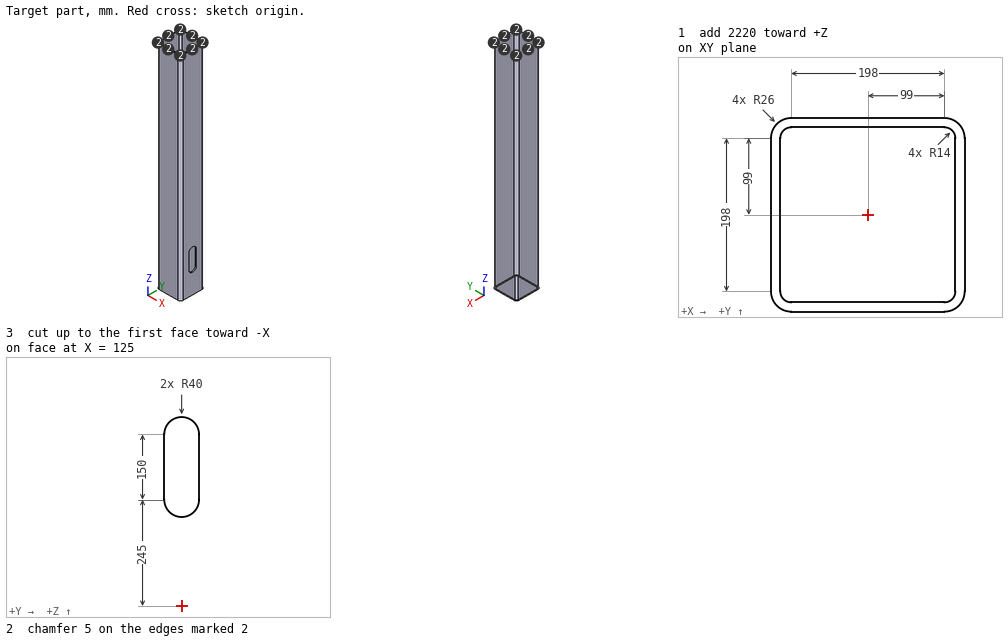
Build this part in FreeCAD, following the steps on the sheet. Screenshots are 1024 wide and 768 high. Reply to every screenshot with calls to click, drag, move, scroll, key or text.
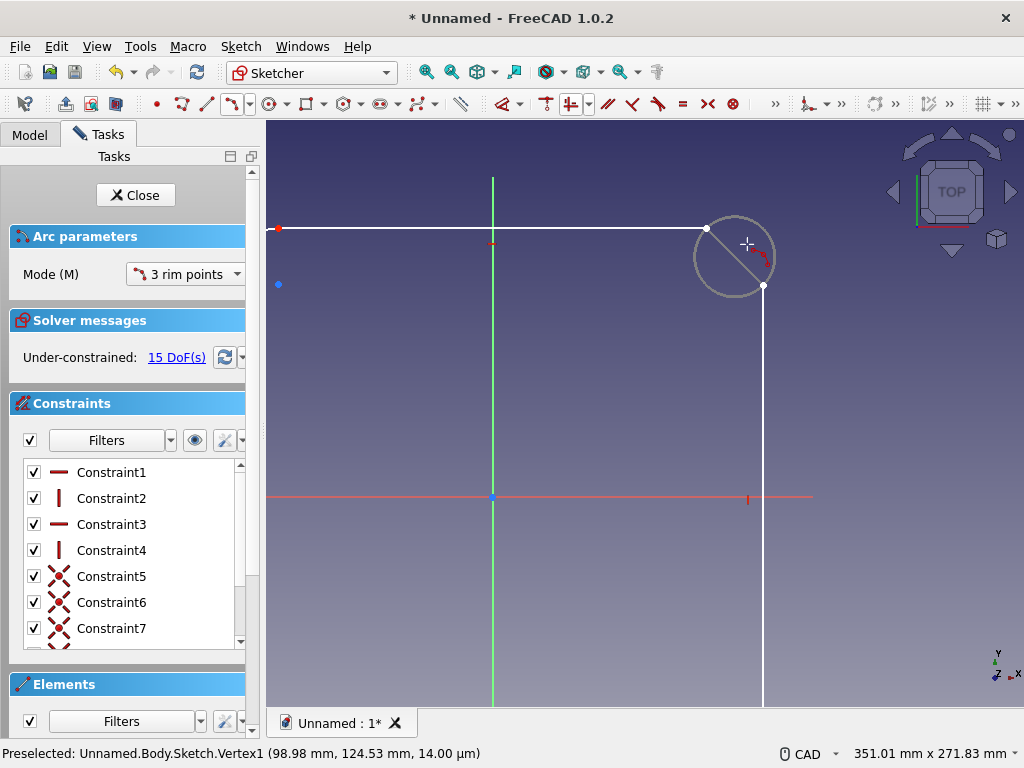
click(746, 244)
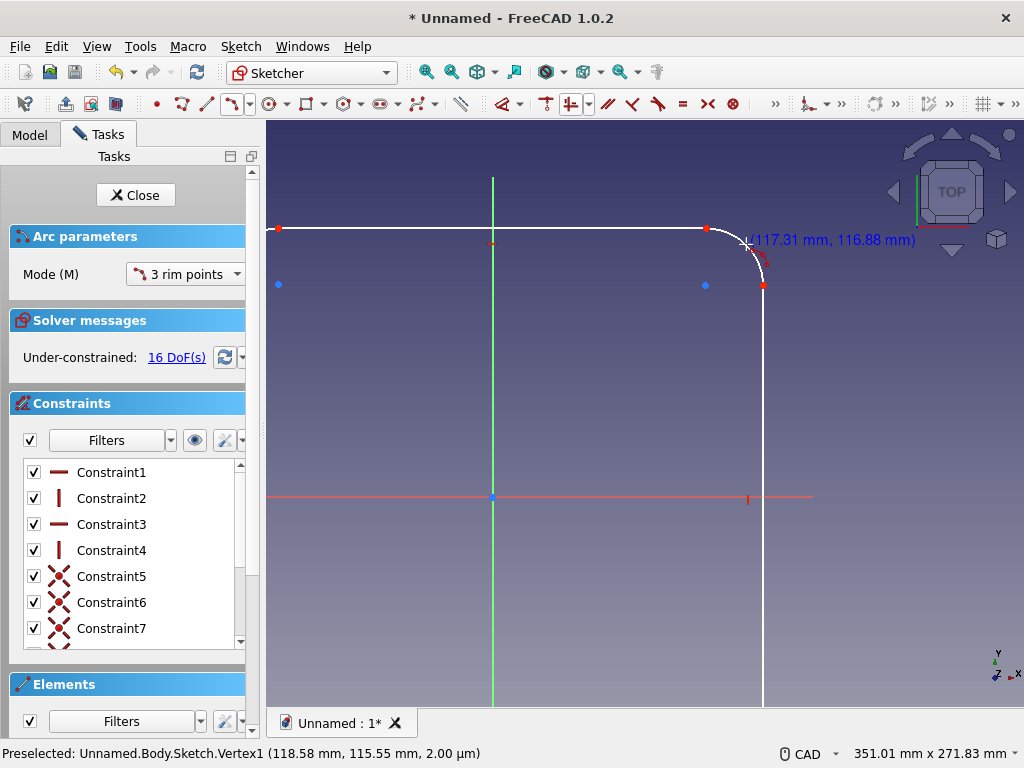
click(207, 104)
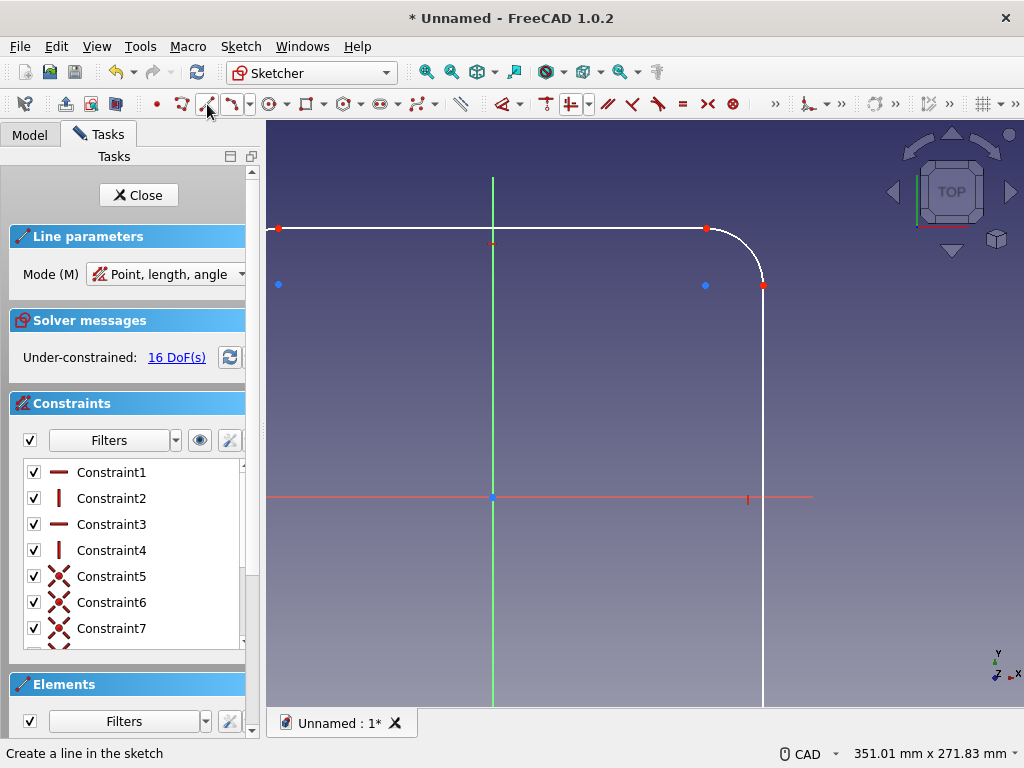
scroll(747, 243, down, 2)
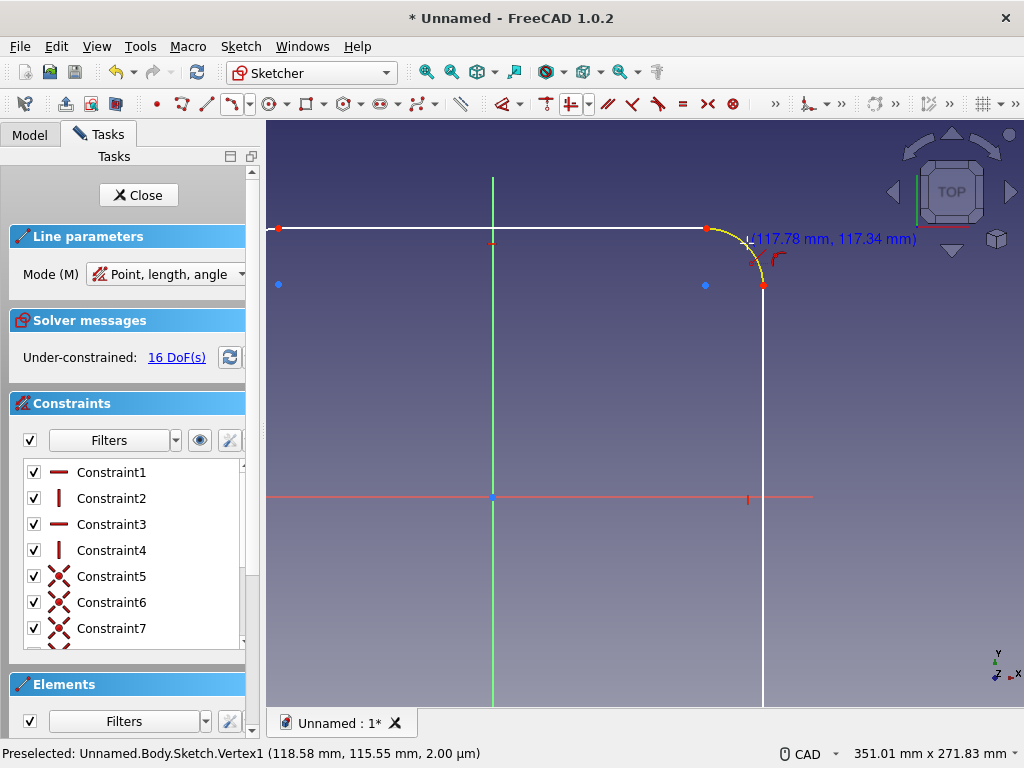
click(433, 250)
click(720, 250)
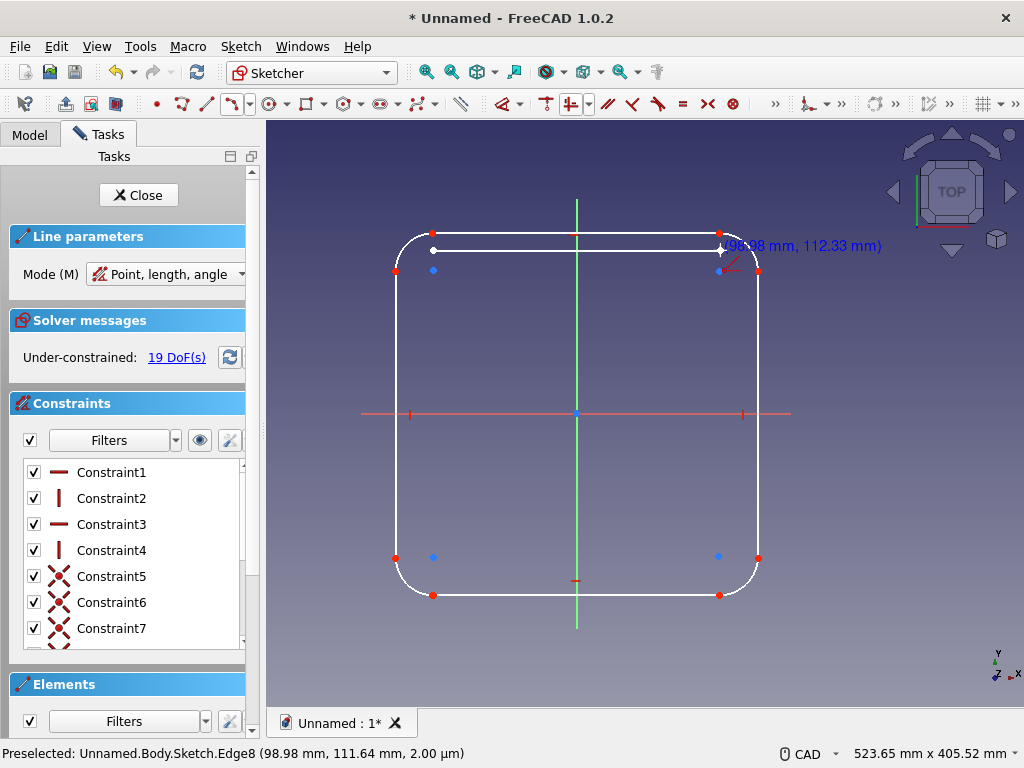
click(740, 270)
click(740, 557)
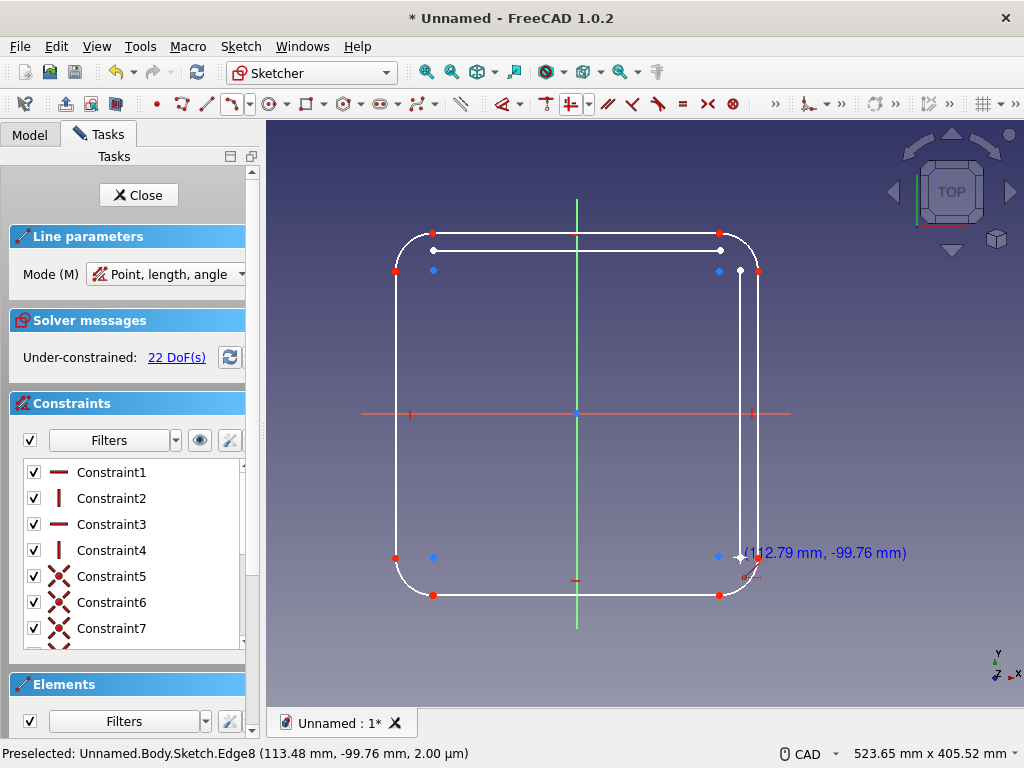
click(720, 577)
click(433, 577)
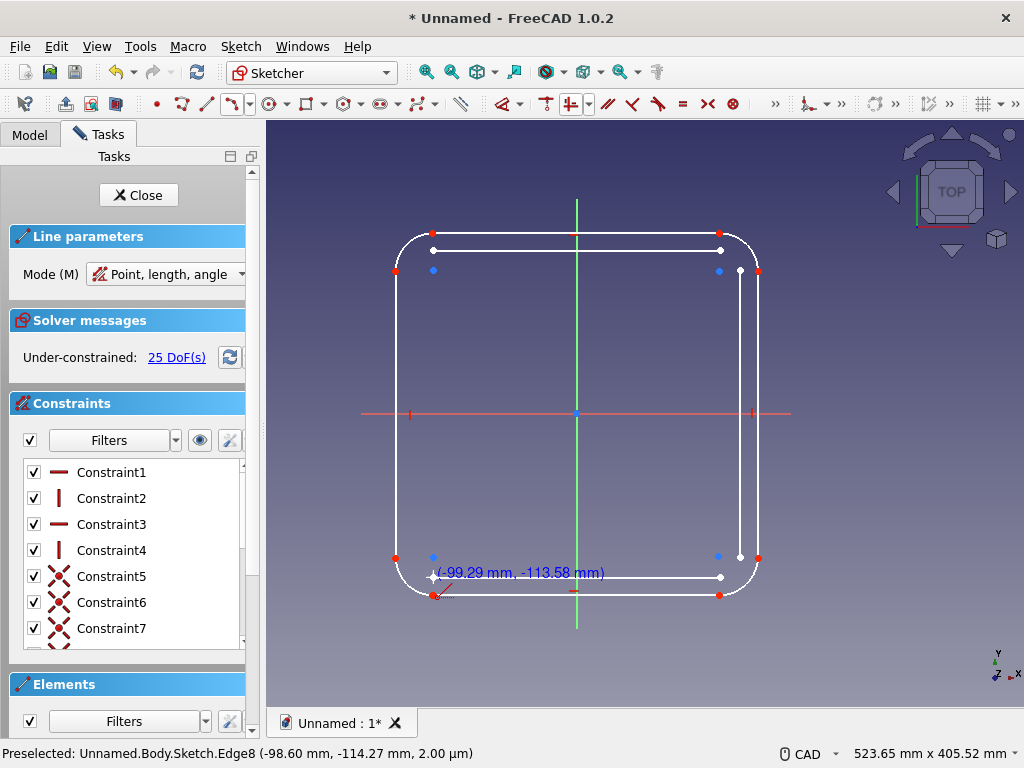
click(413, 557)
click(413, 270)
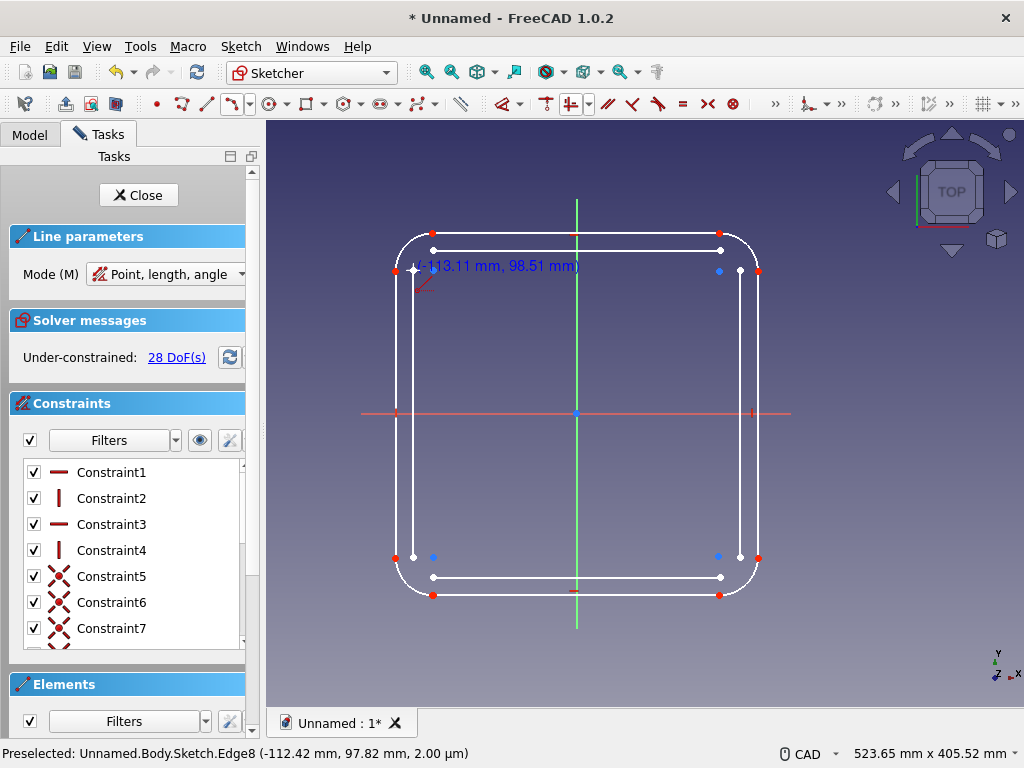
click(232, 104)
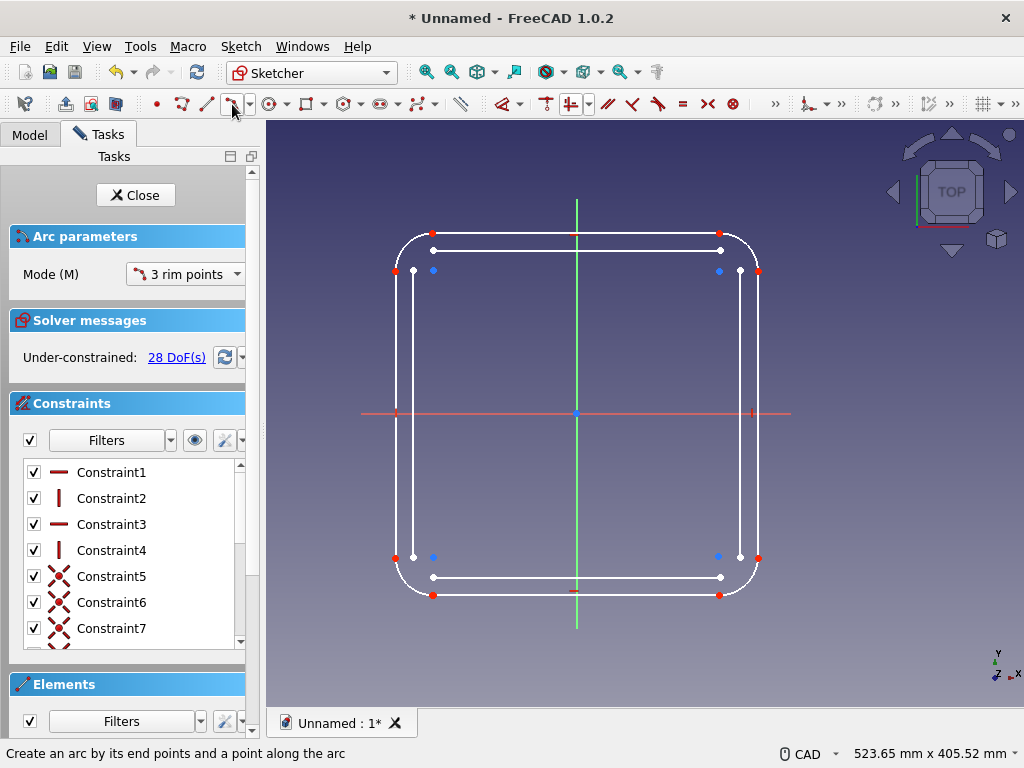
click(720, 251)
click(740, 271)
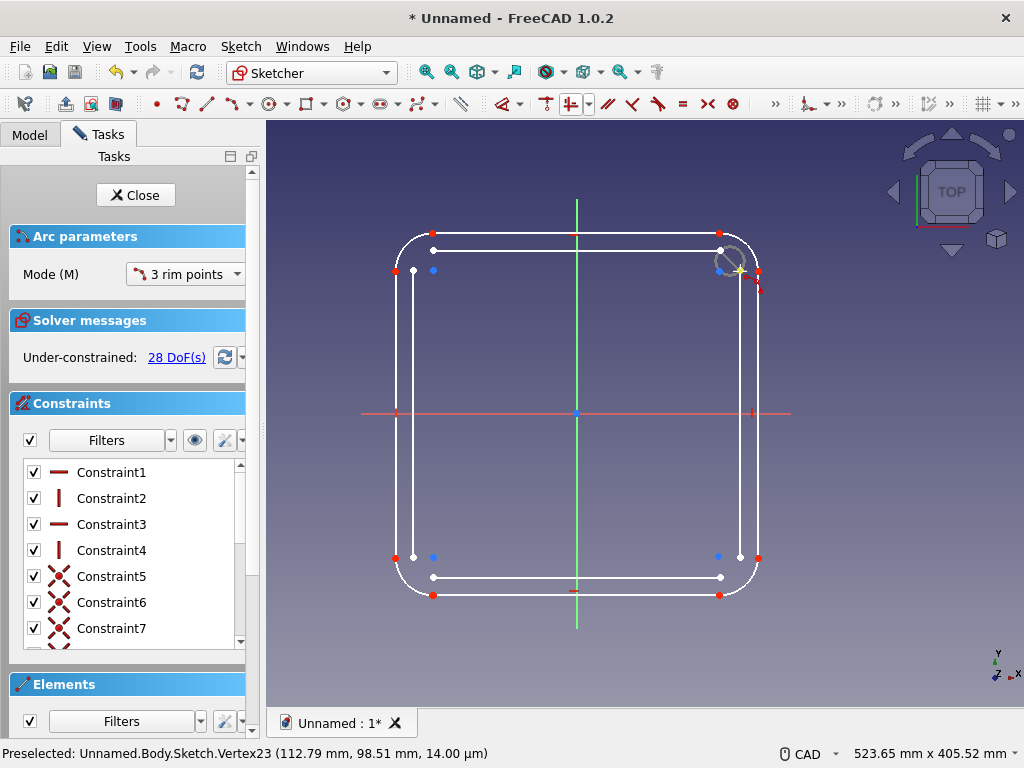
scroll(734, 256, up, 5)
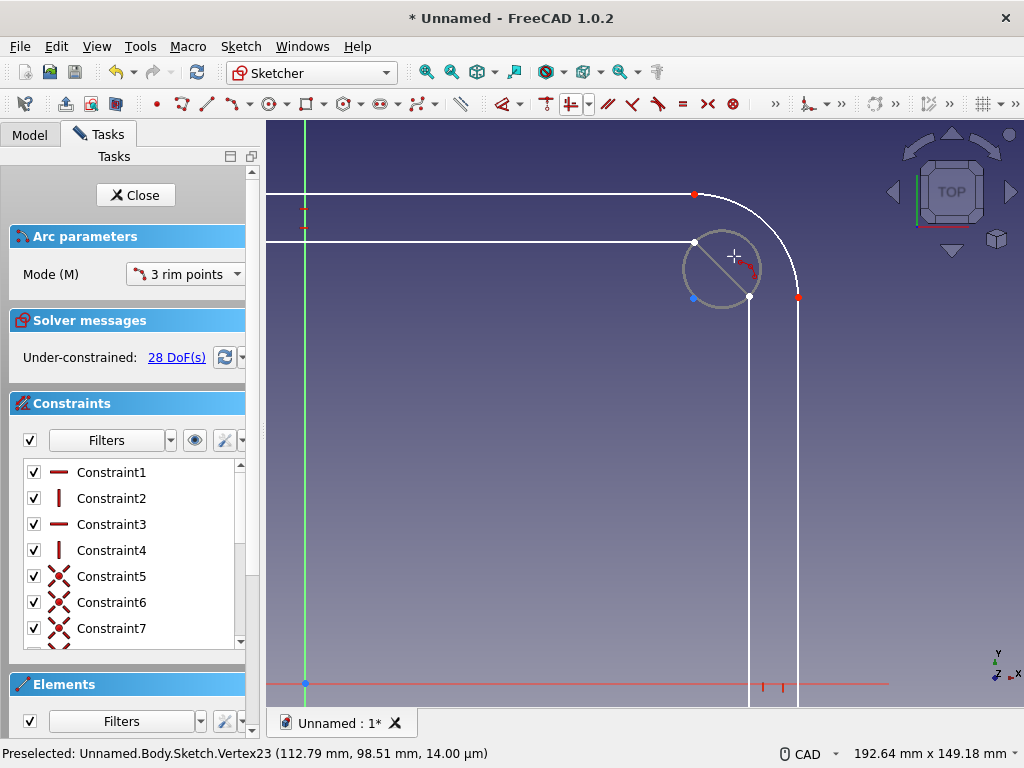
click(734, 255)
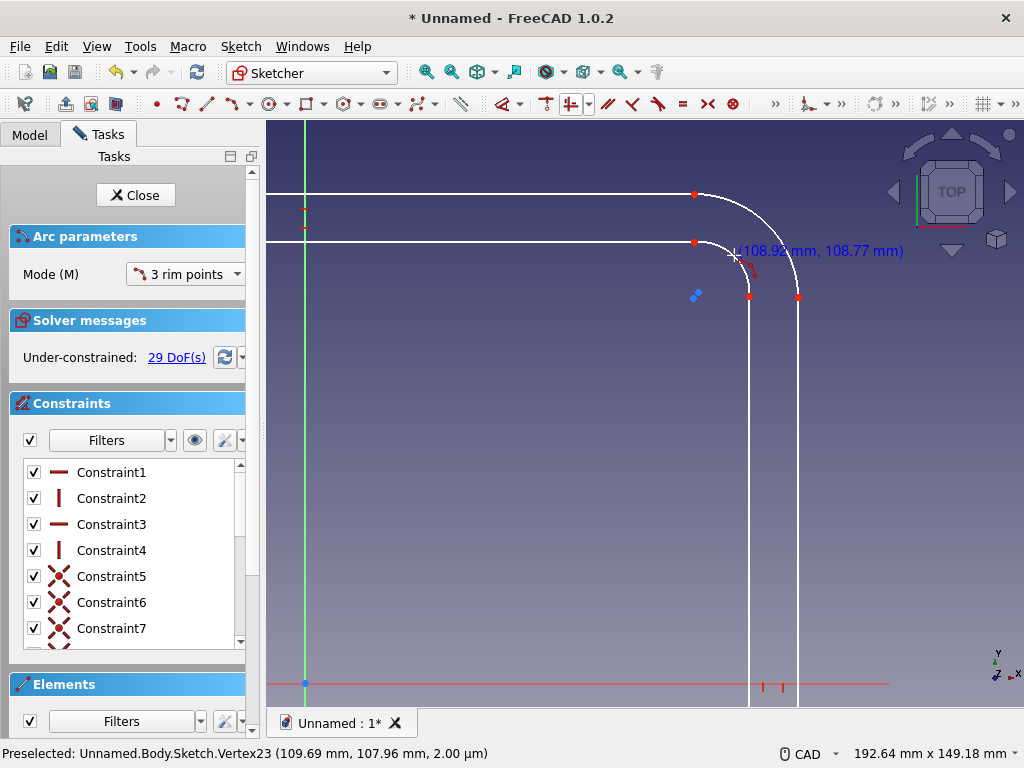
scroll(734, 256, down, 5)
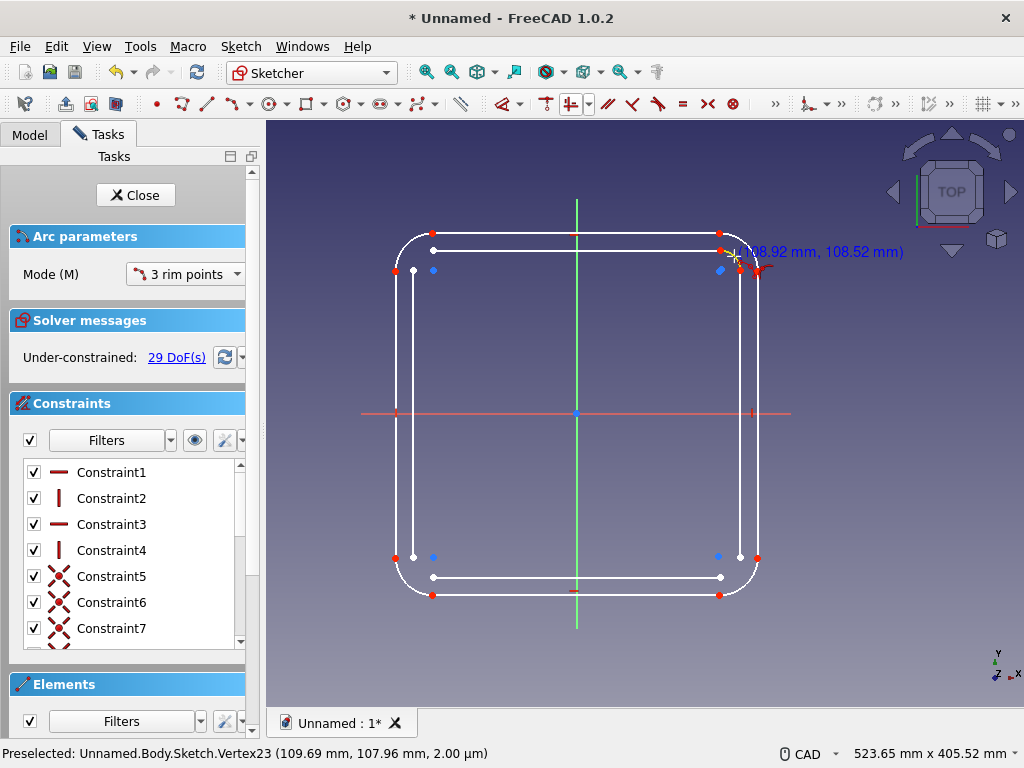
click(740, 558)
click(720, 578)